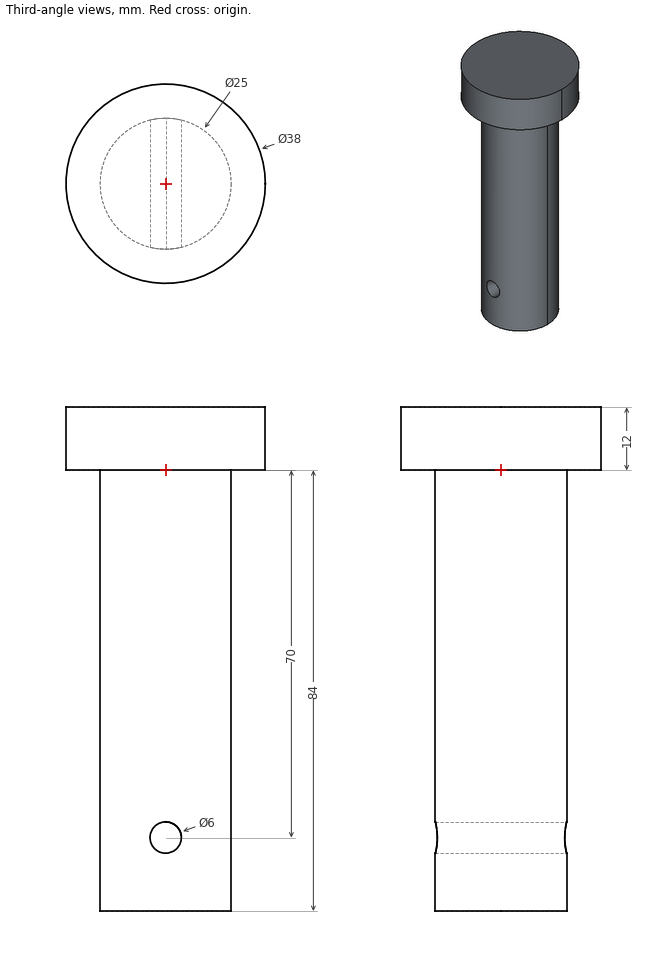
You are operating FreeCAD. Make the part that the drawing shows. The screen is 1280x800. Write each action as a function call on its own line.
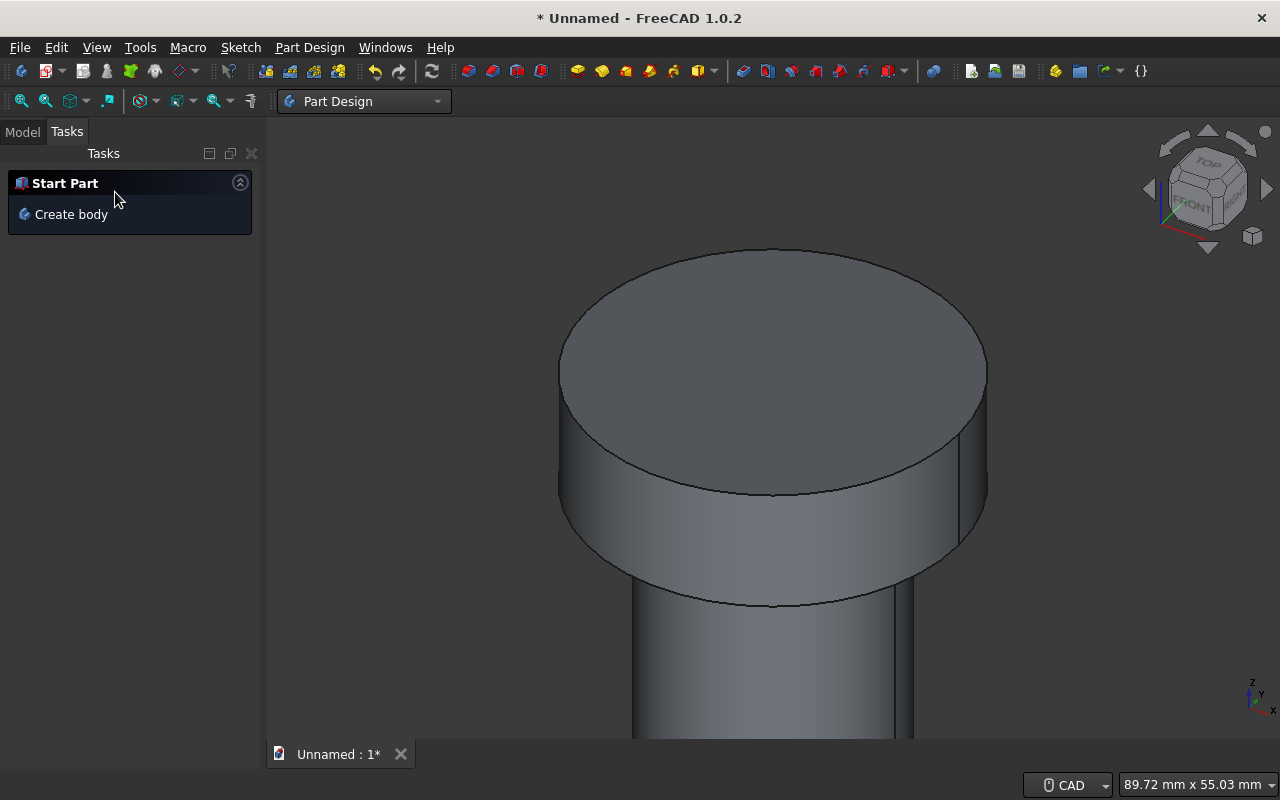
click(22, 102)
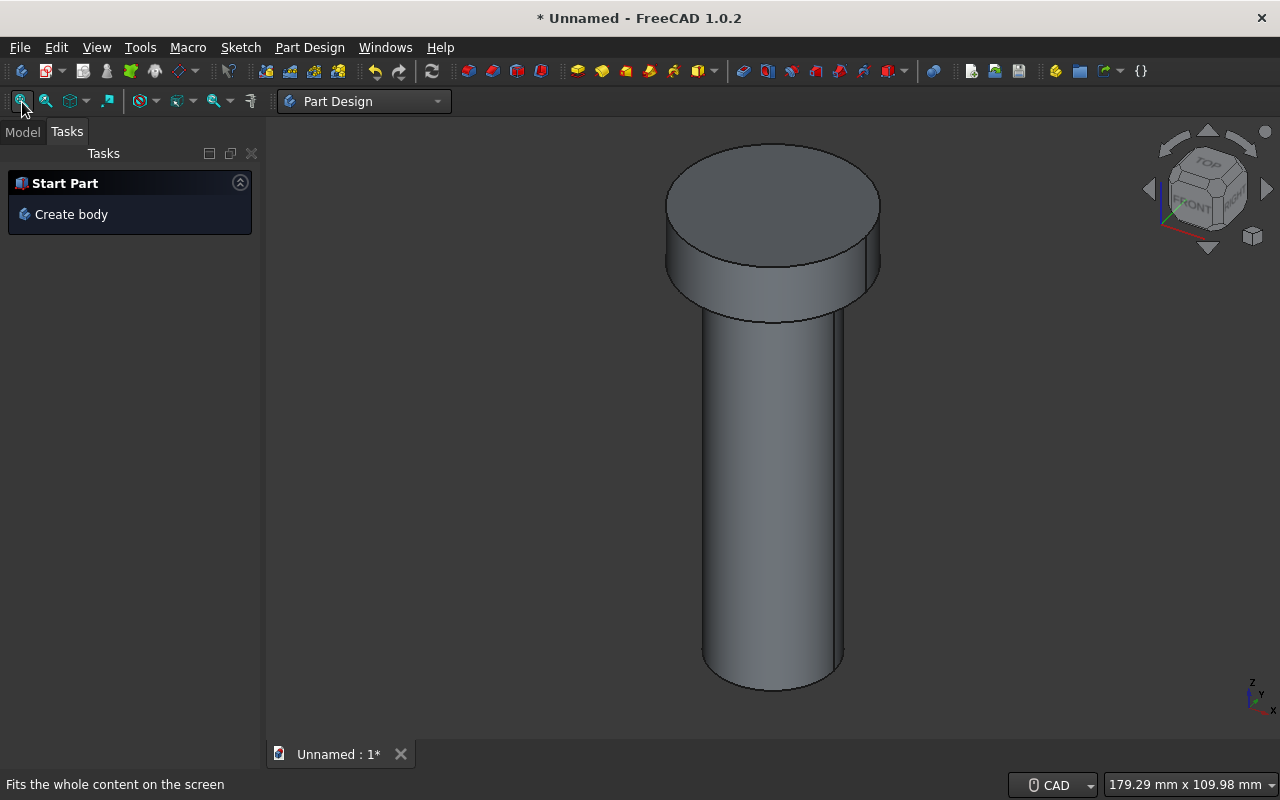
click(46, 72)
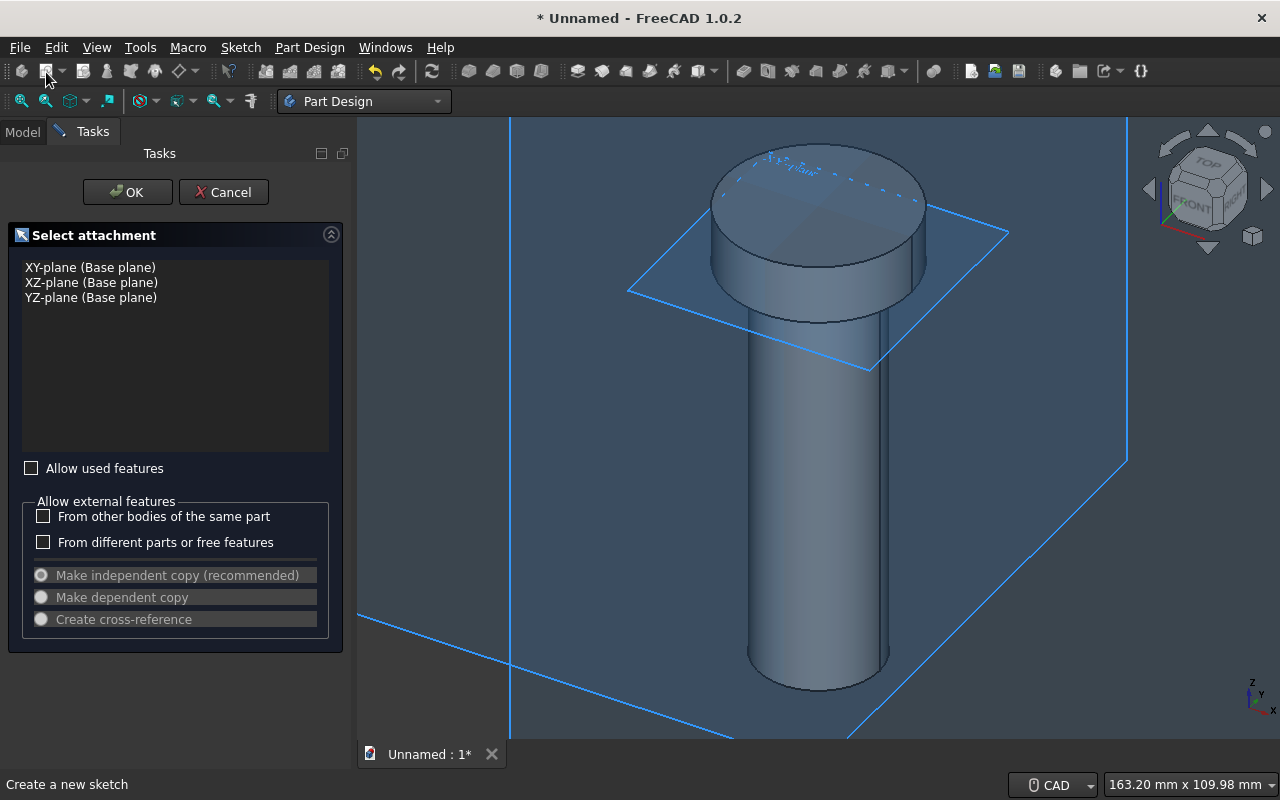
click(82, 282)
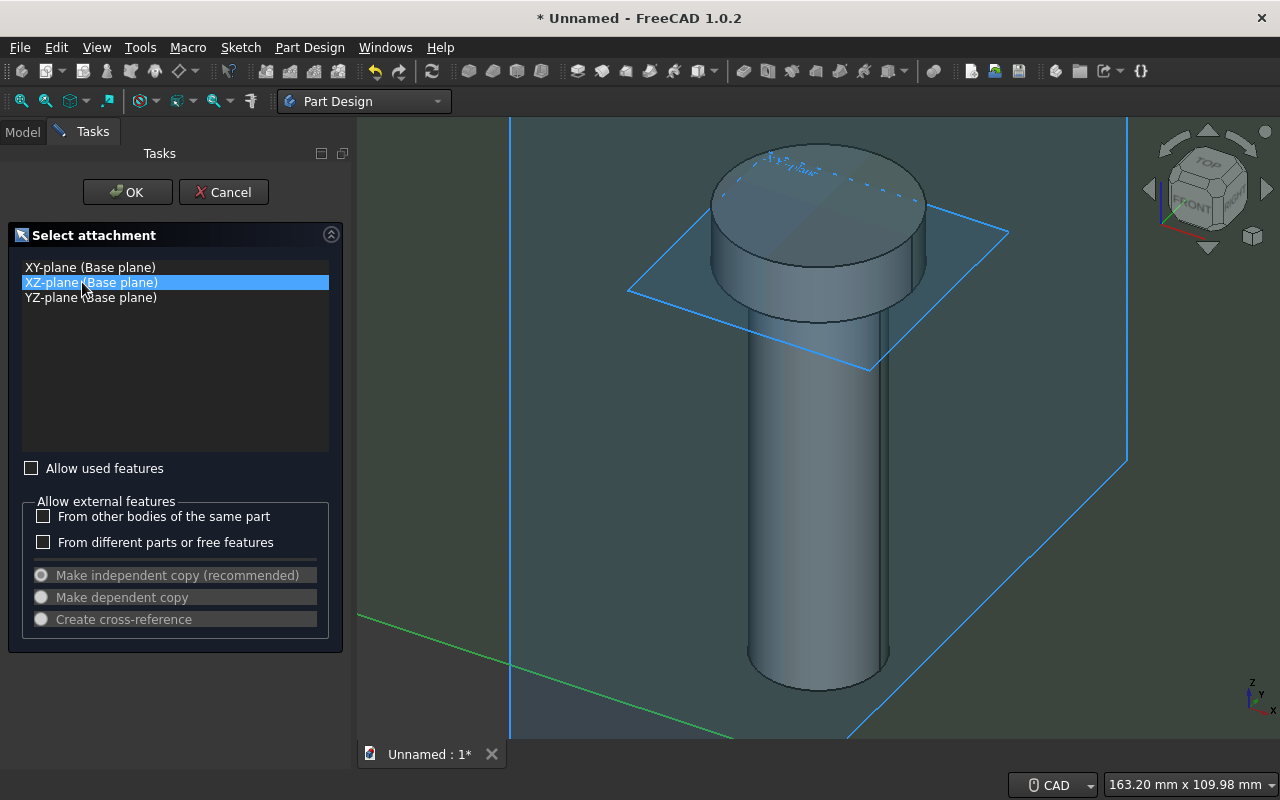
click(128, 192)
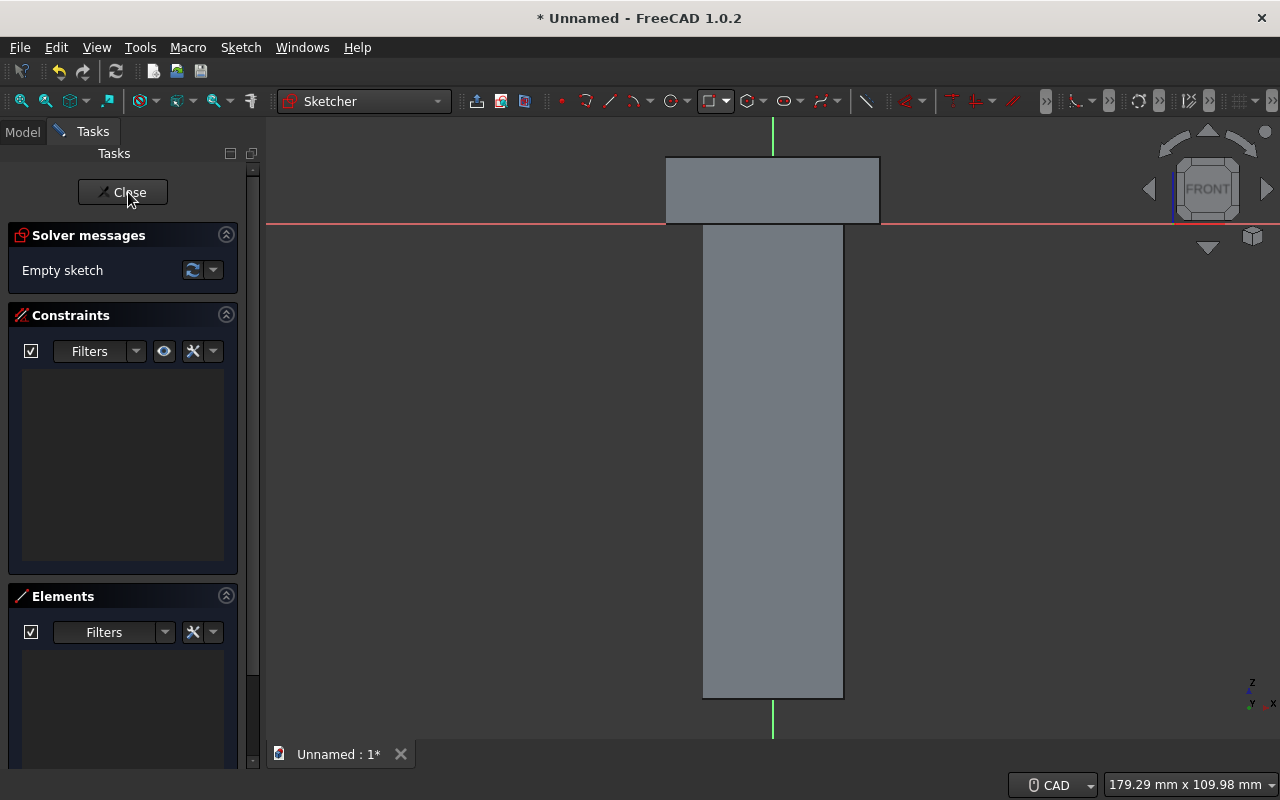
key(q)
key(s)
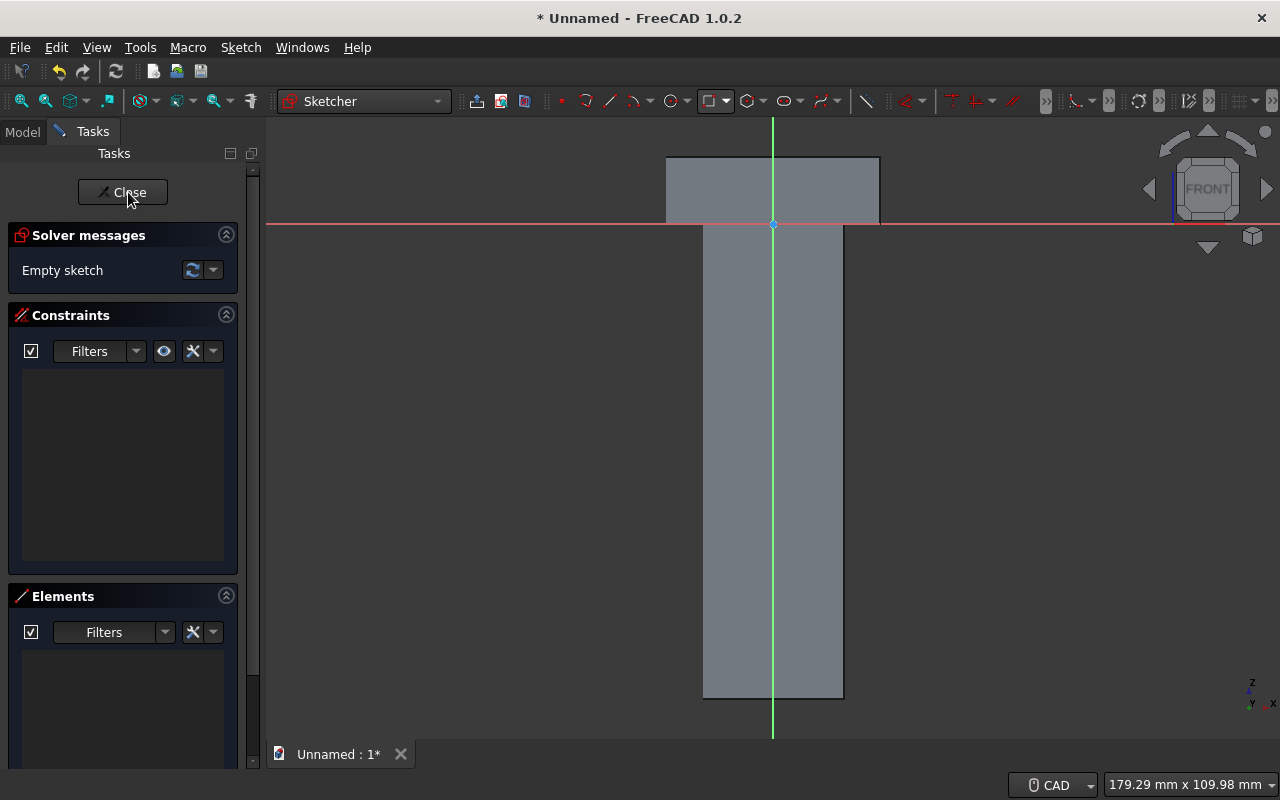
scroll(780, 639, up, 12)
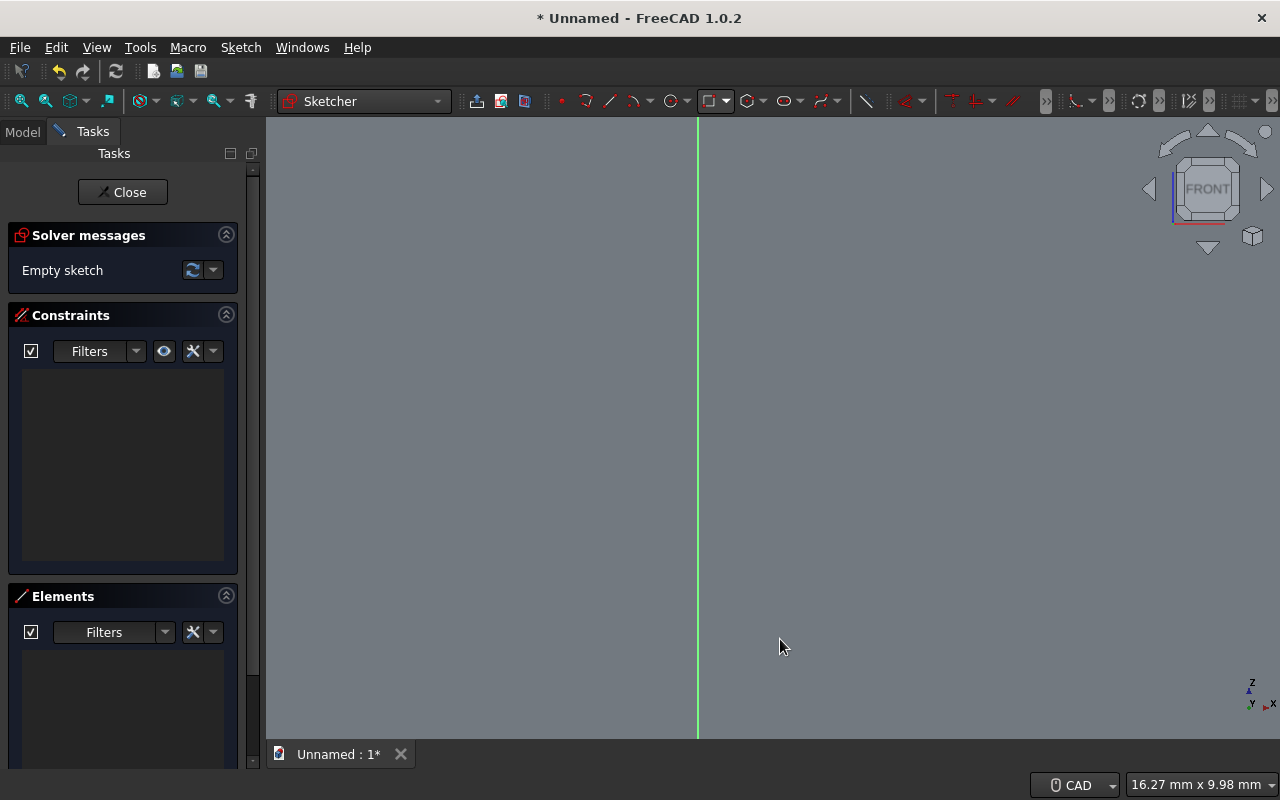
click(672, 102)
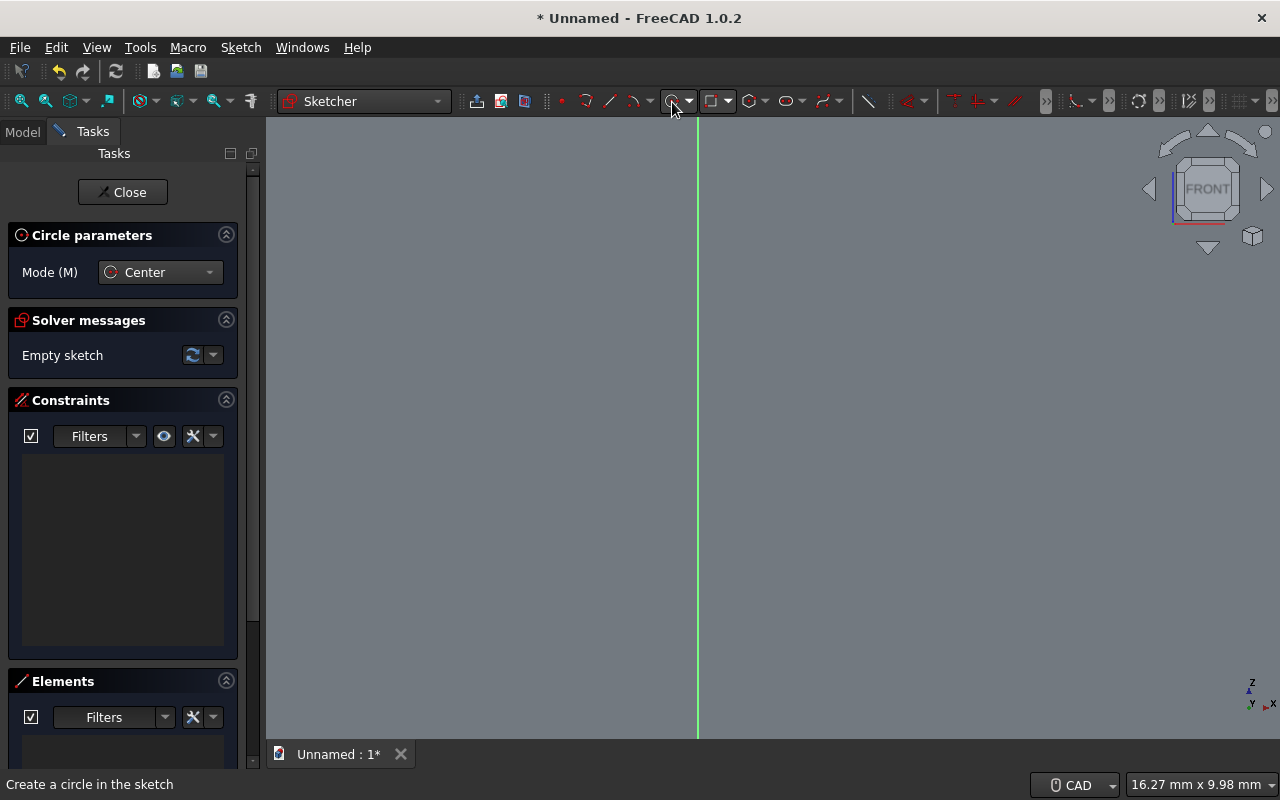
click(698, 424)
click(830, 292)
key(Escape)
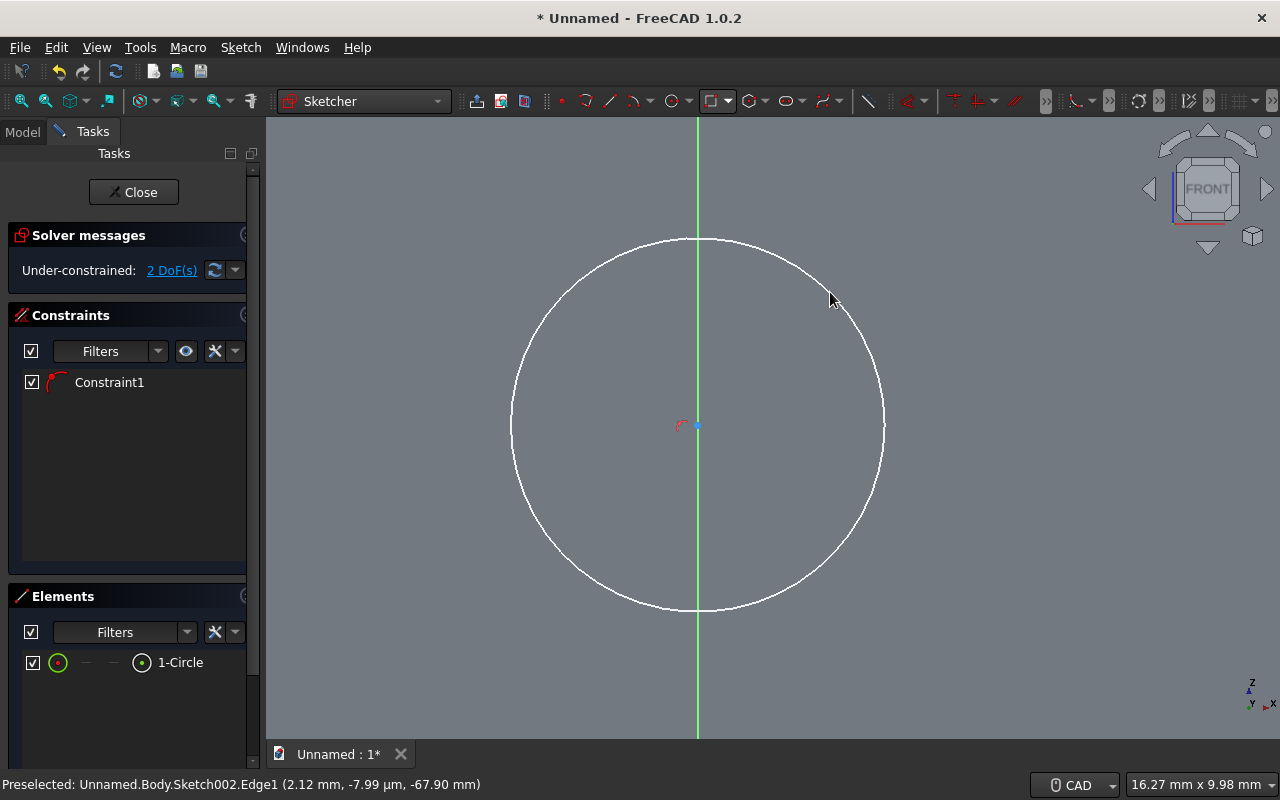
click(908, 102)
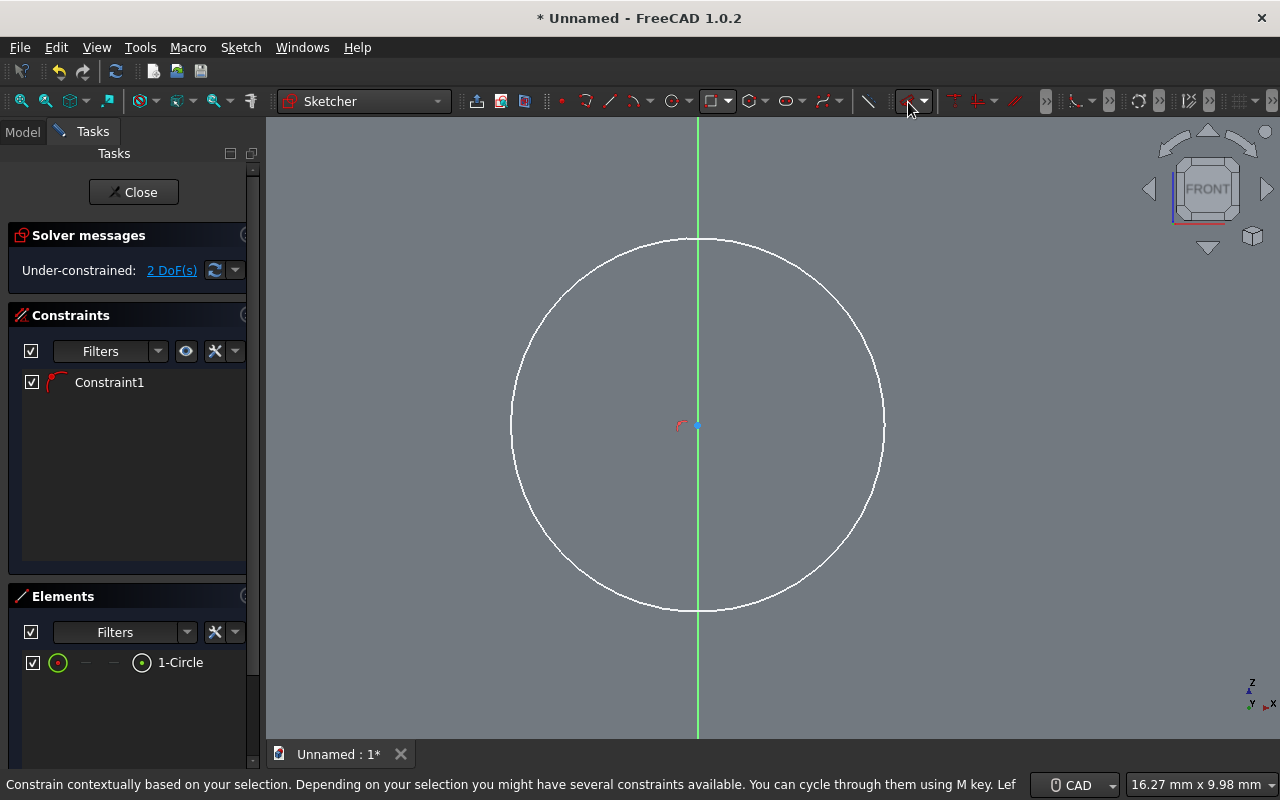
click(829, 292)
click(851, 269)